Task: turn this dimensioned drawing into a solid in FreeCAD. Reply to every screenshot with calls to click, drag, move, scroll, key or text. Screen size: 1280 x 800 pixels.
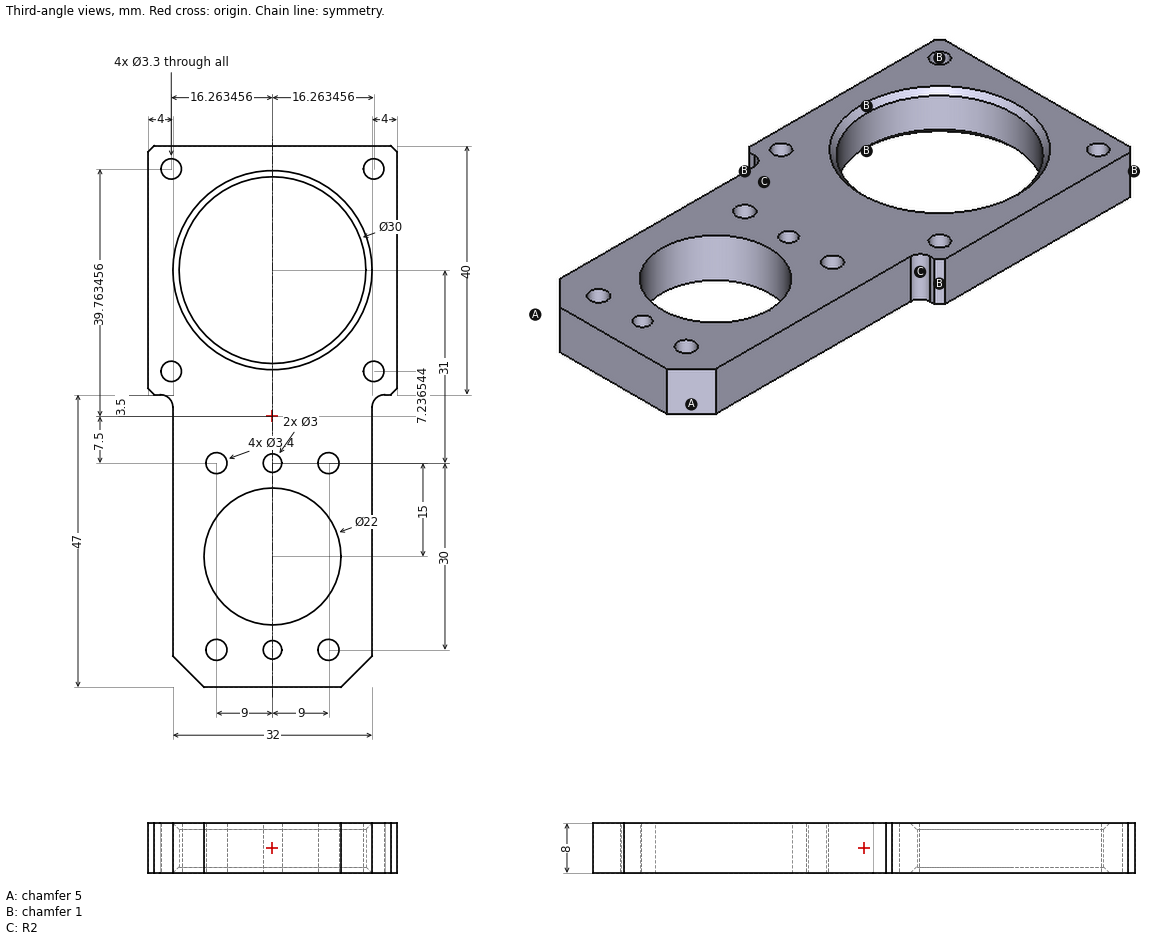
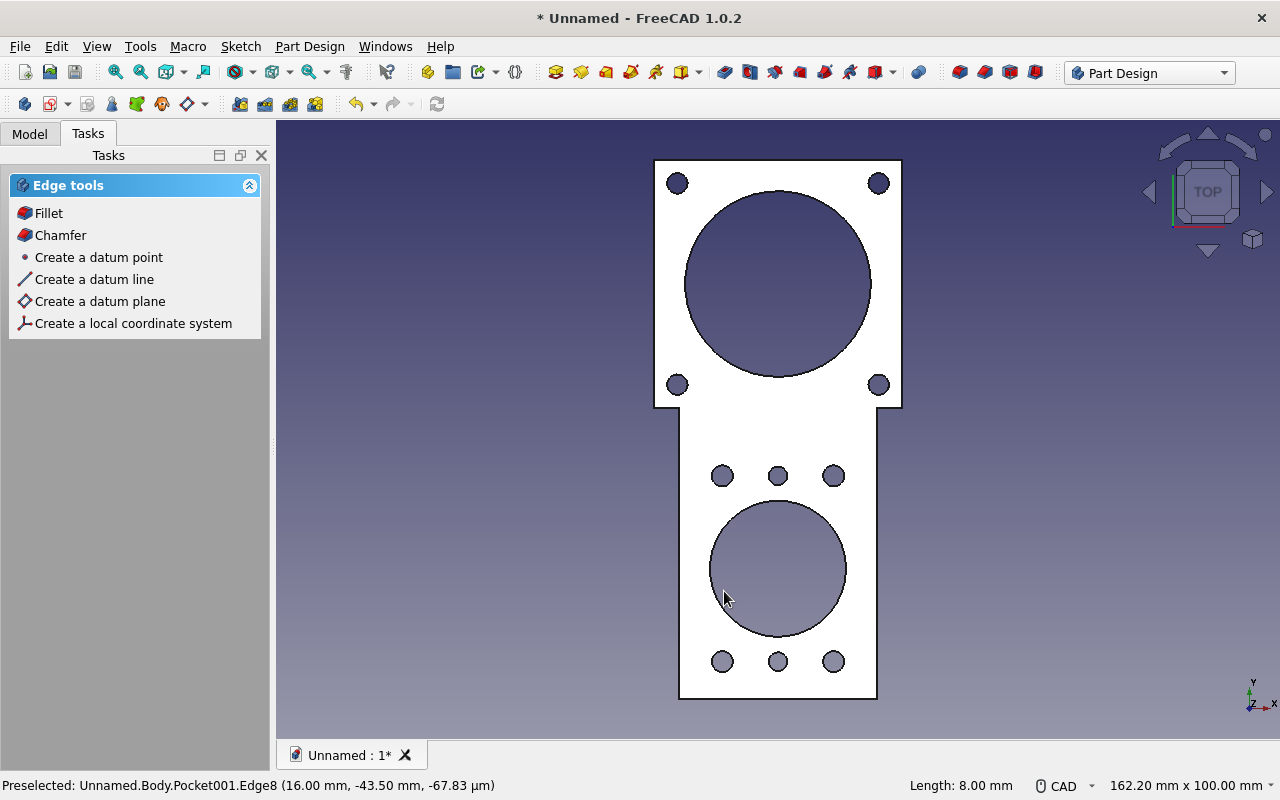
key(1)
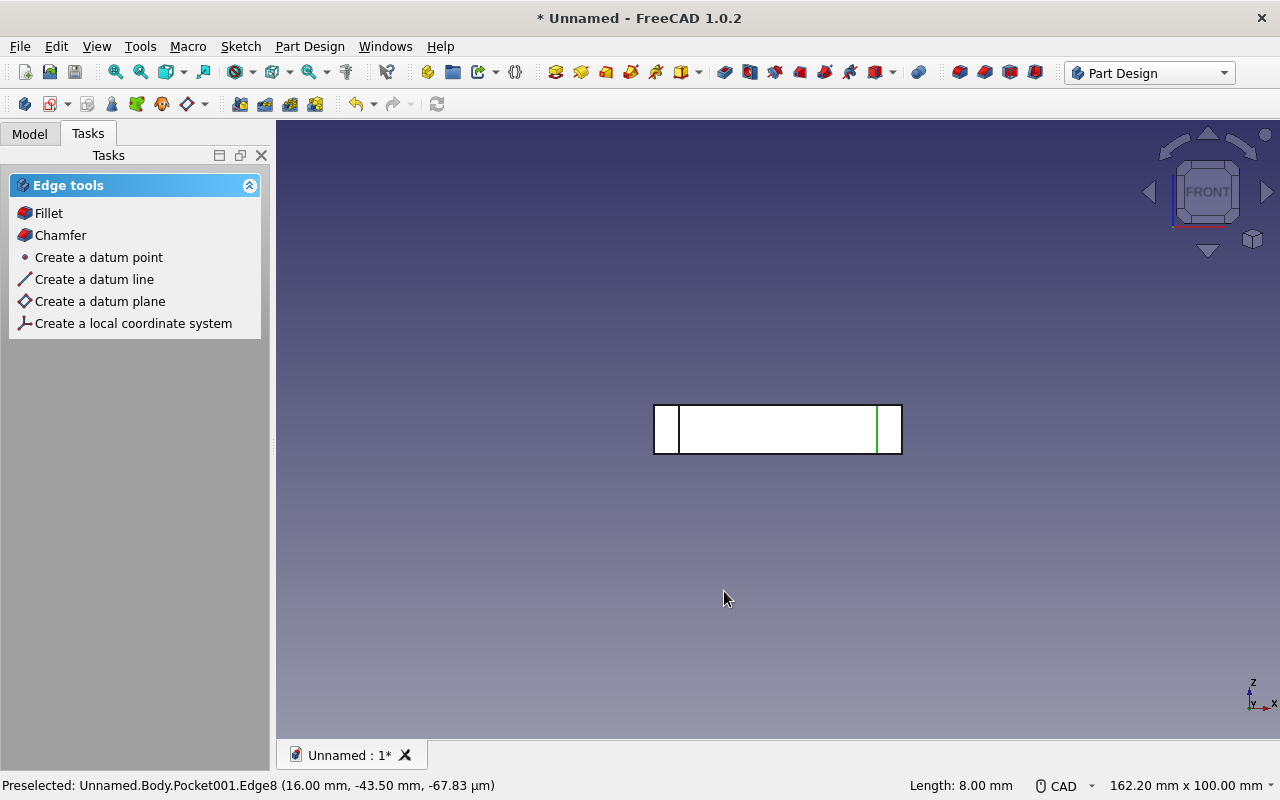
click(116, 72)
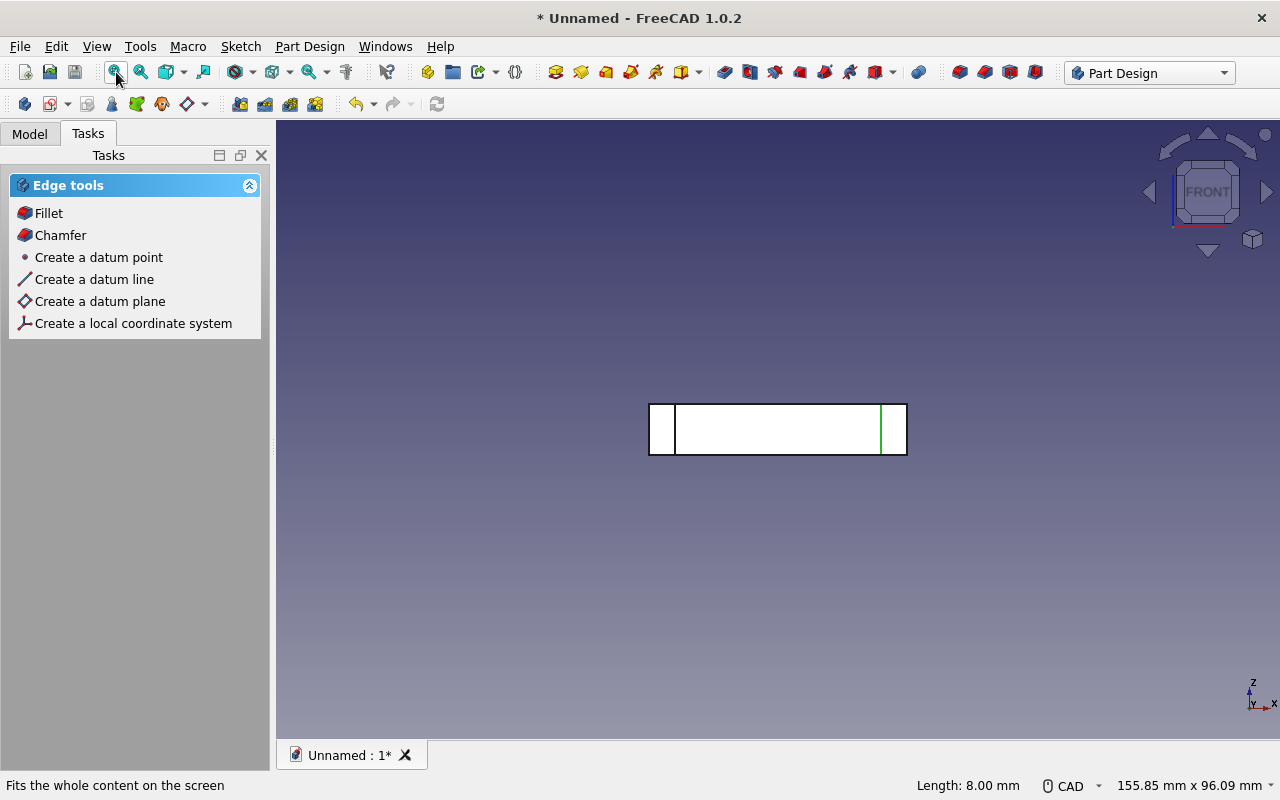
click(675, 429, ctrl)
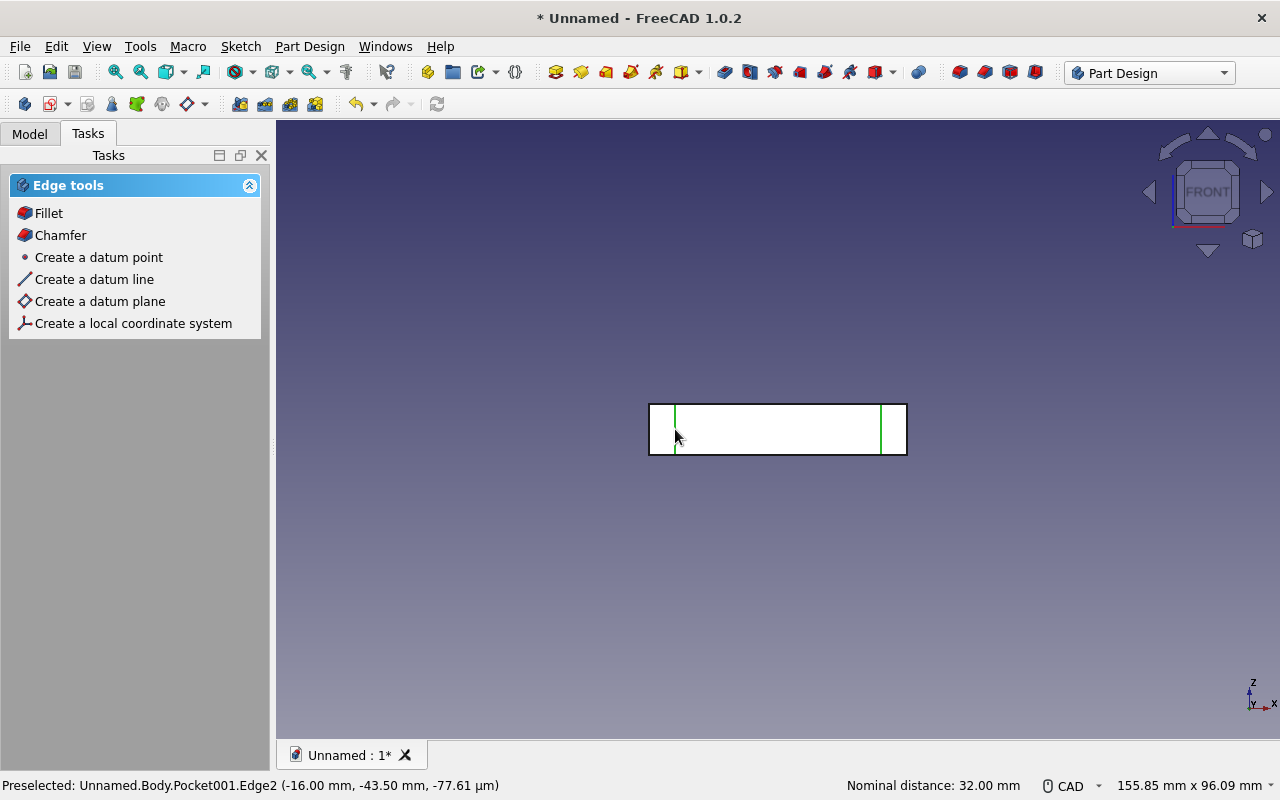
click(985, 72)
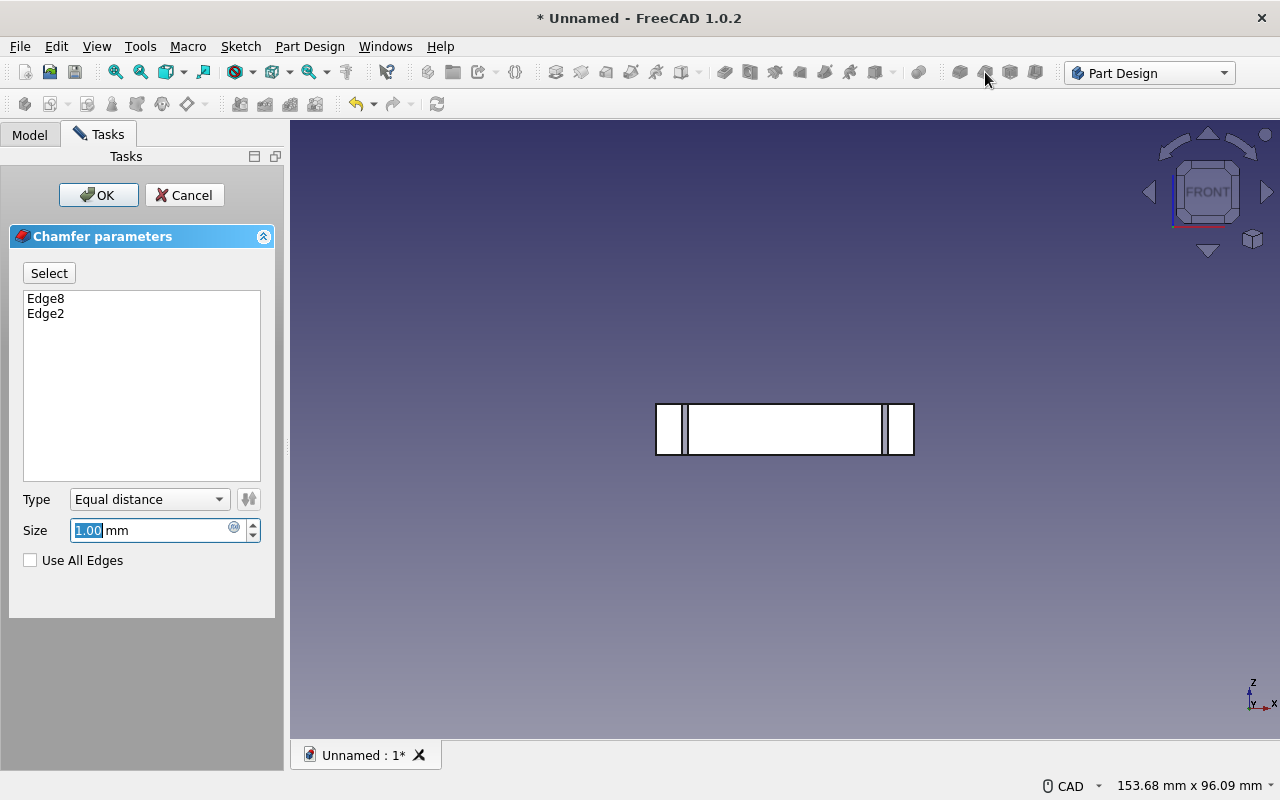
text(5)
key(Tab)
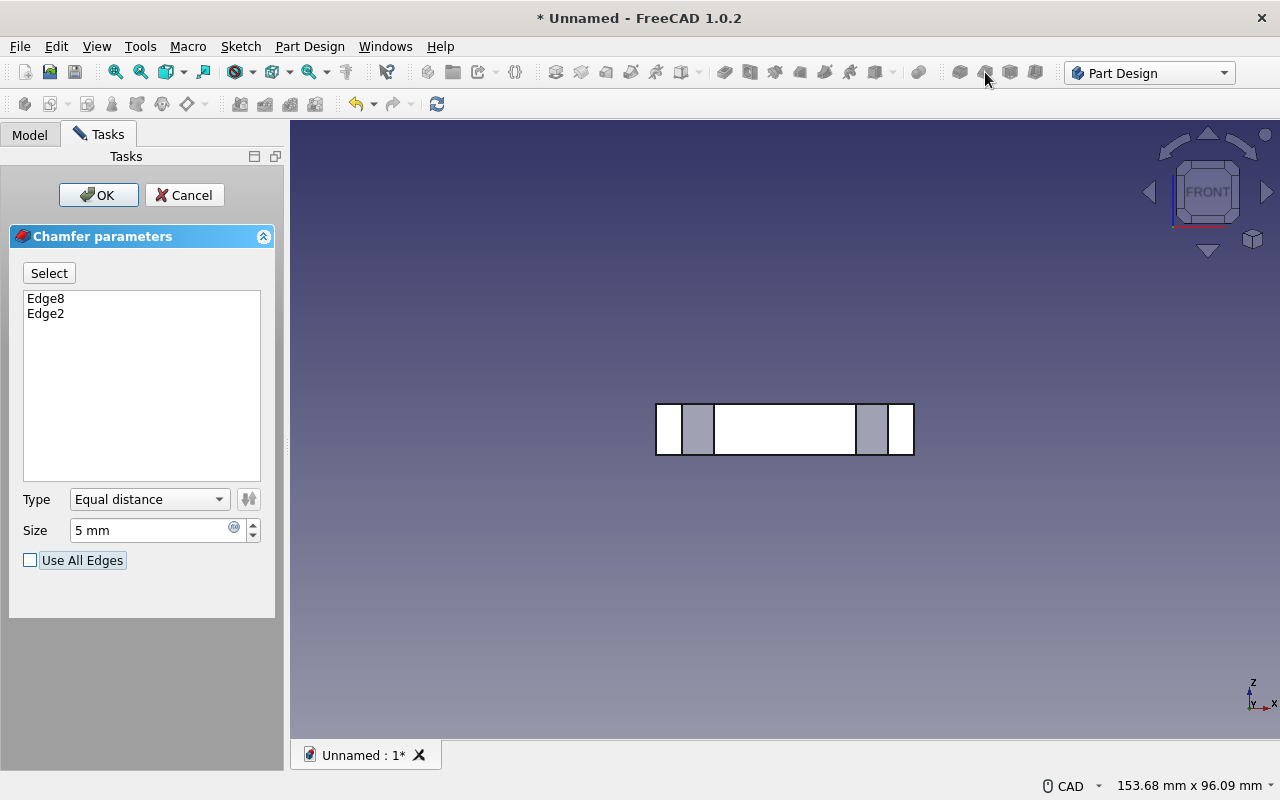
click(99, 195)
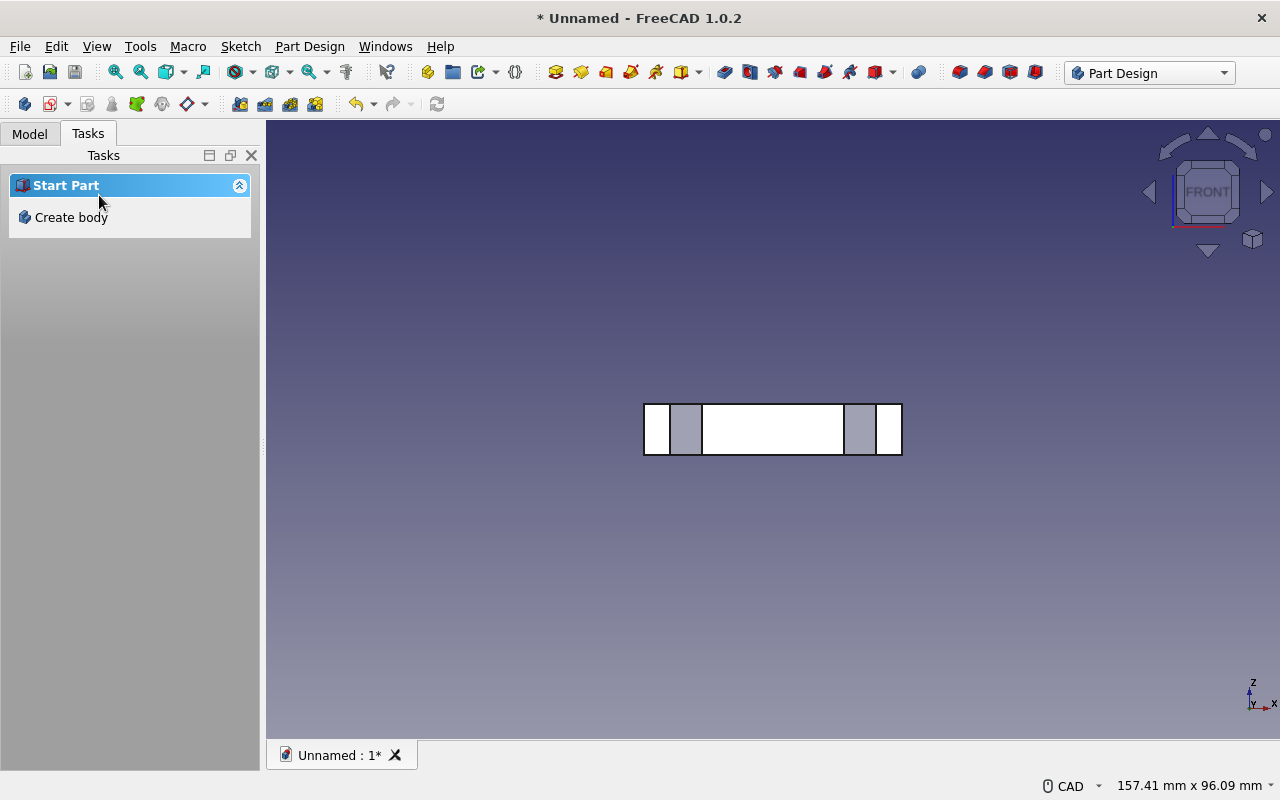
click(116, 72)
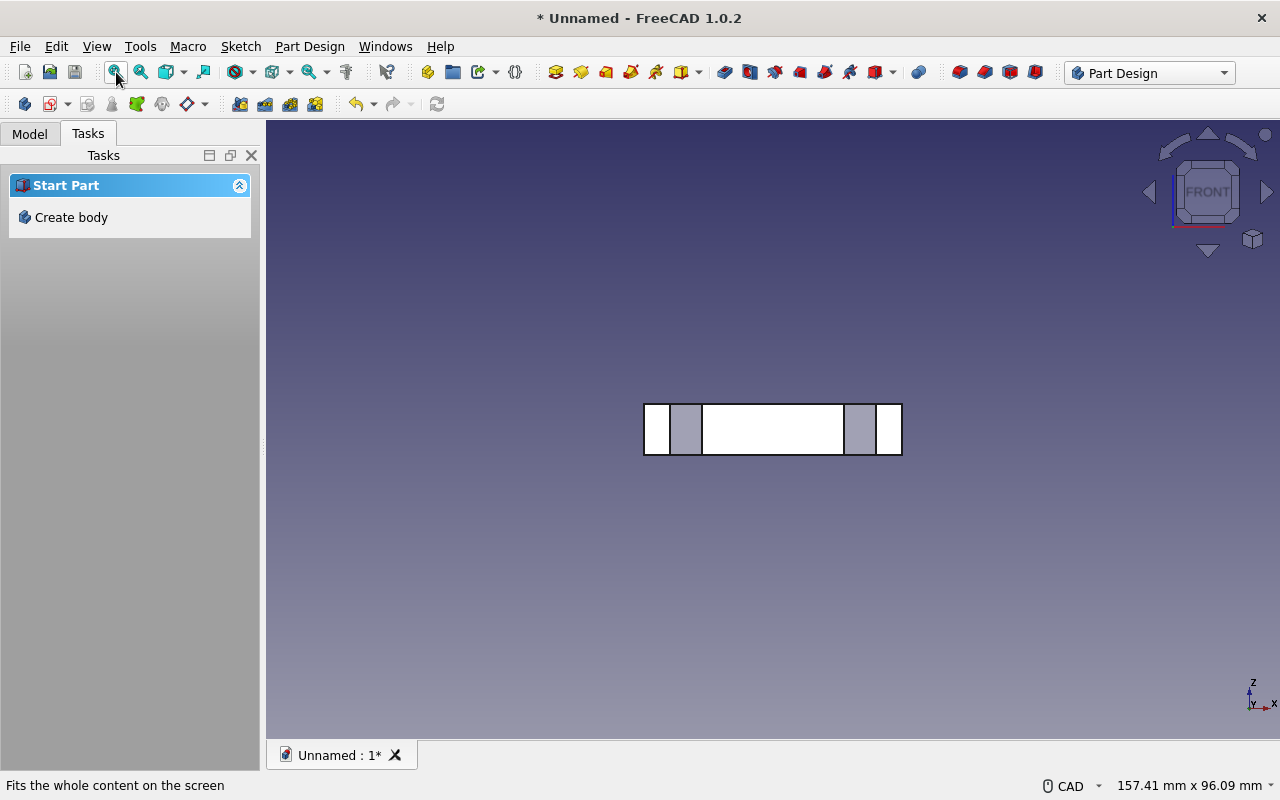
click(644, 429)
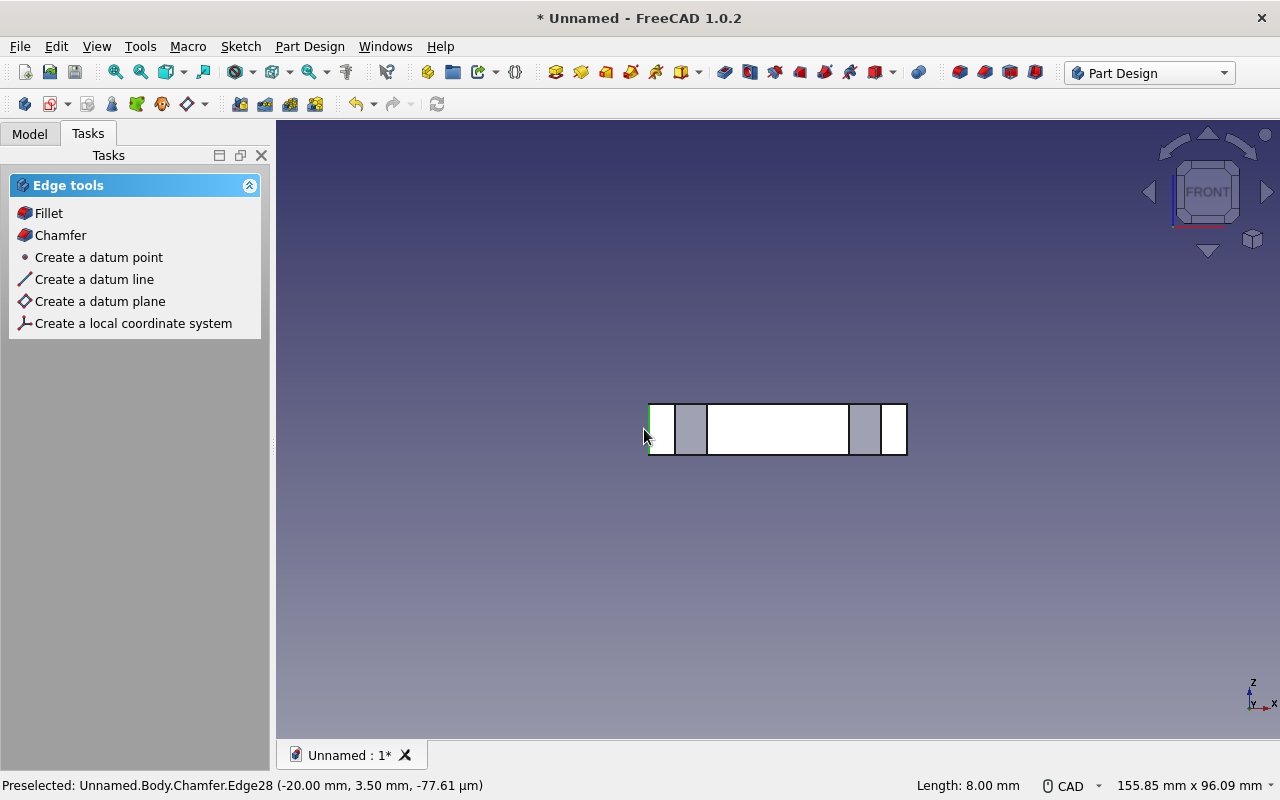
click(907, 429, ctrl)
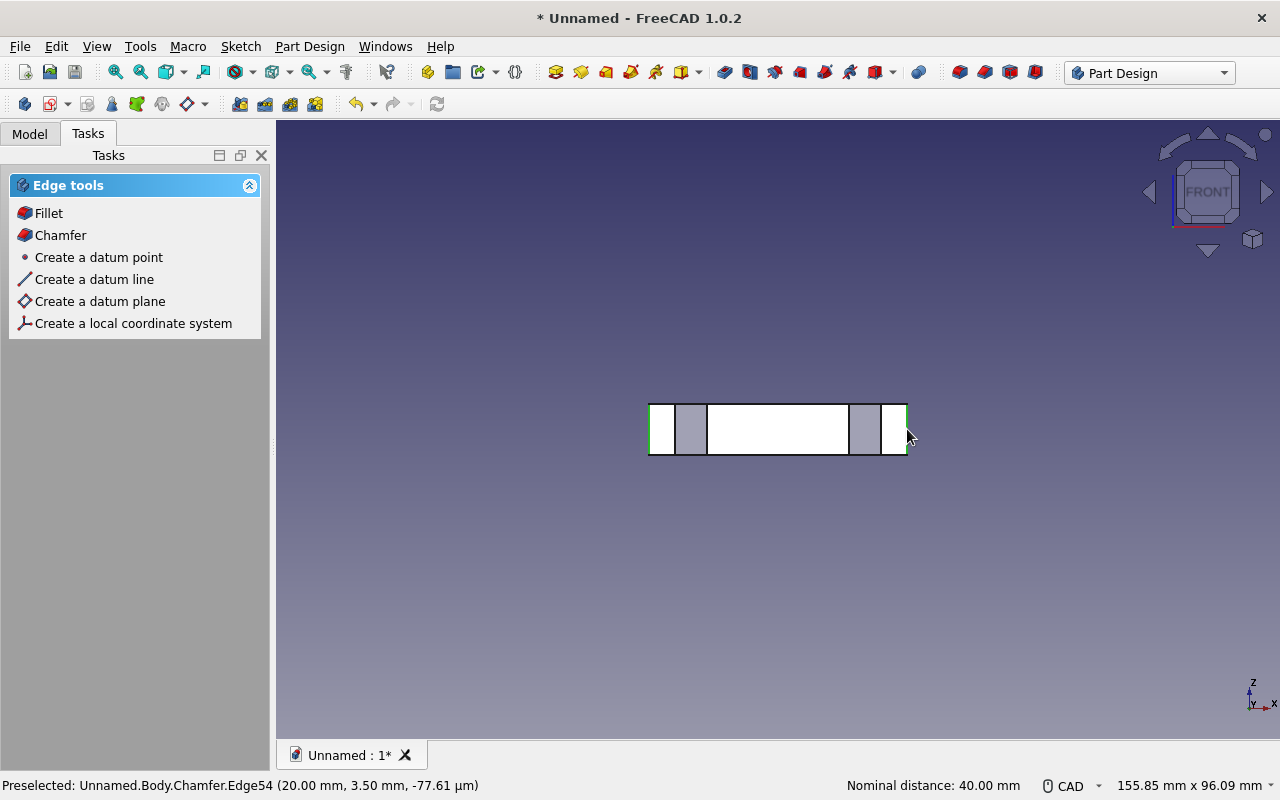
key(0)